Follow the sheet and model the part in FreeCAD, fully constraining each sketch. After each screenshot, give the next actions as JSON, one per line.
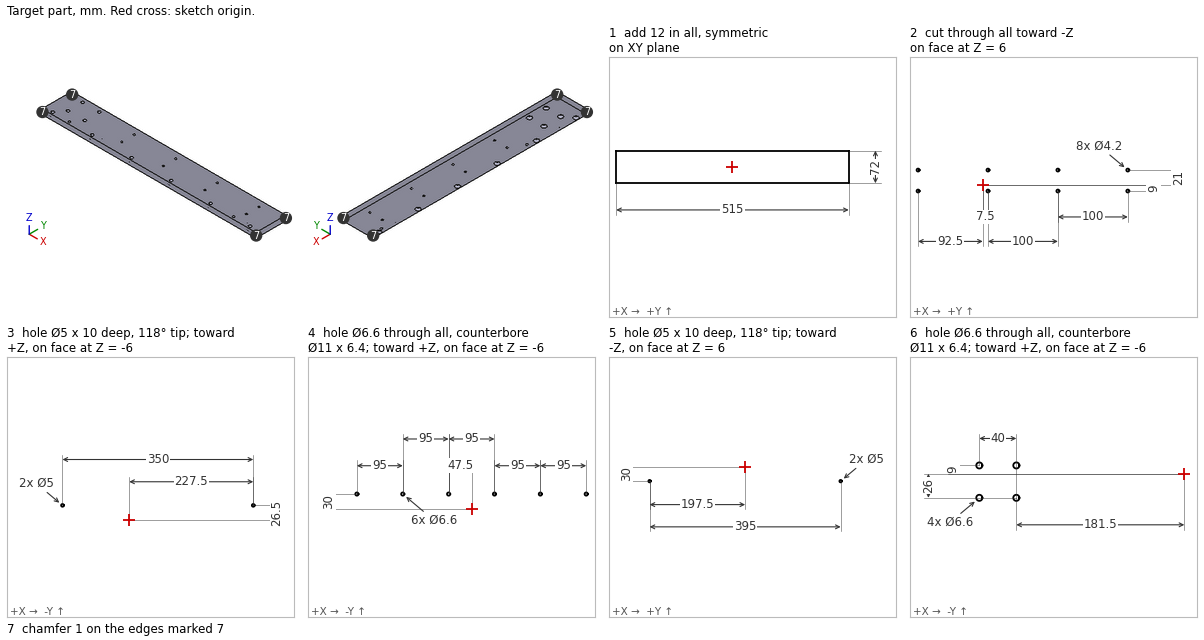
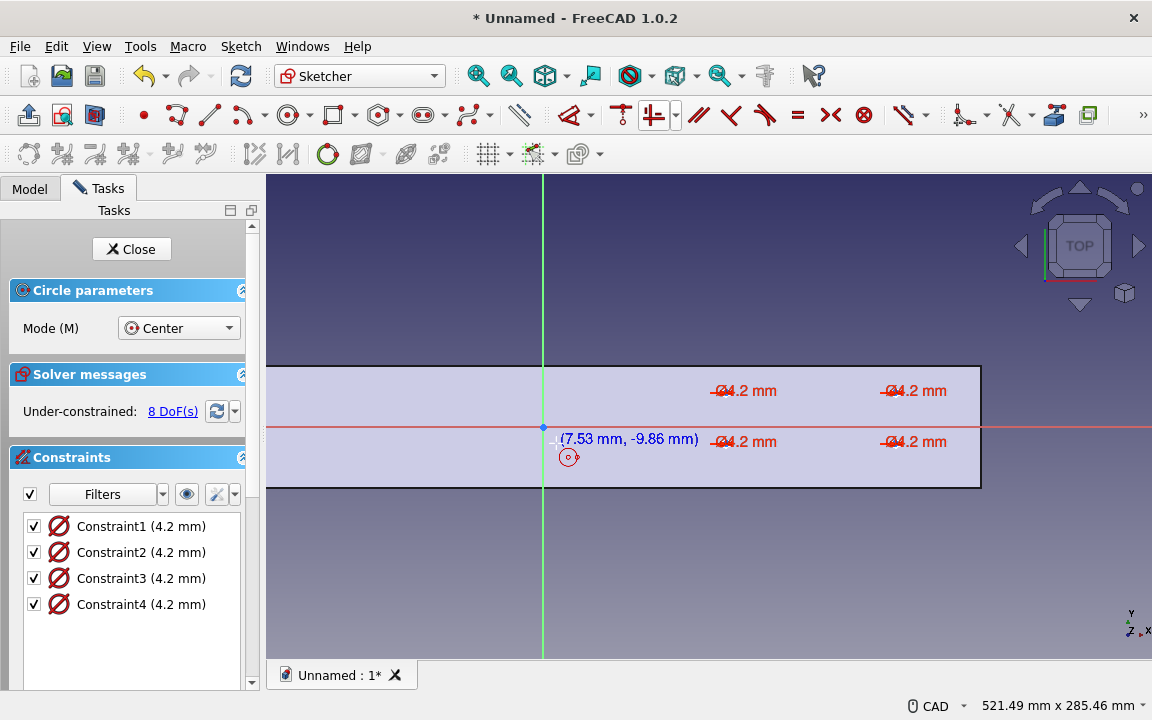
{"action": "scroll", "coordinate": [556, 443], "scroll_direction": "up", "scroll_amount": 2}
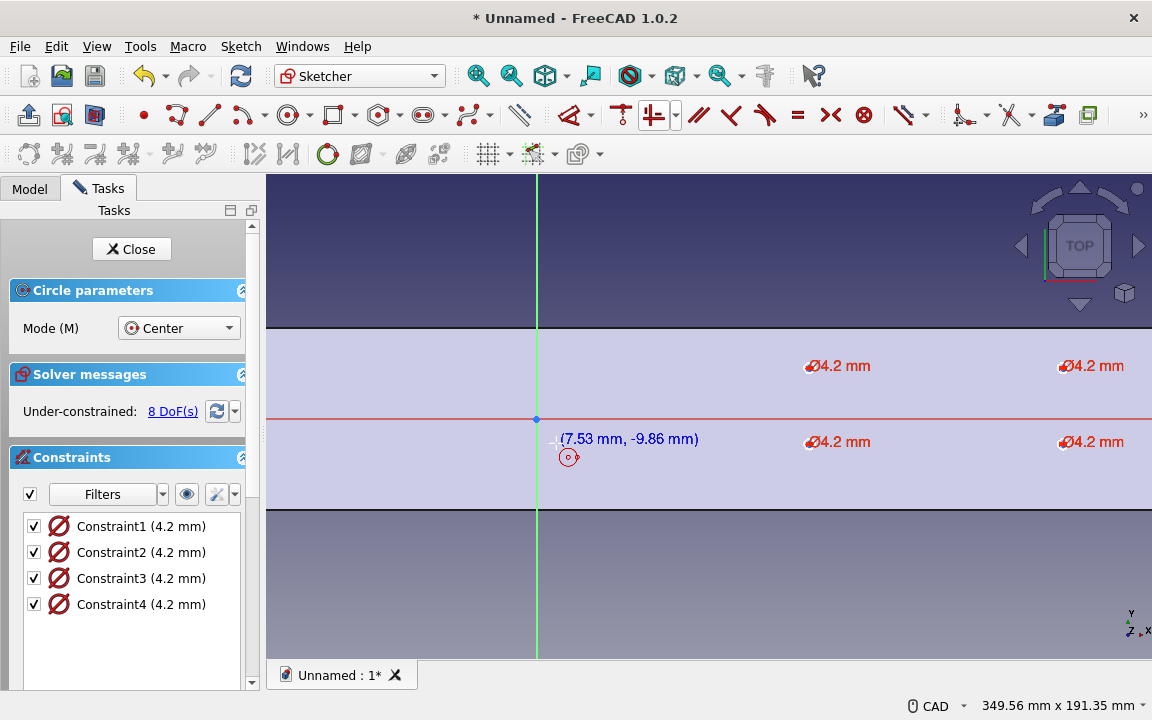
{"action": "left_click", "coordinate": [556, 442]}
{"action": "mouse_move", "coordinate": [560, 438]}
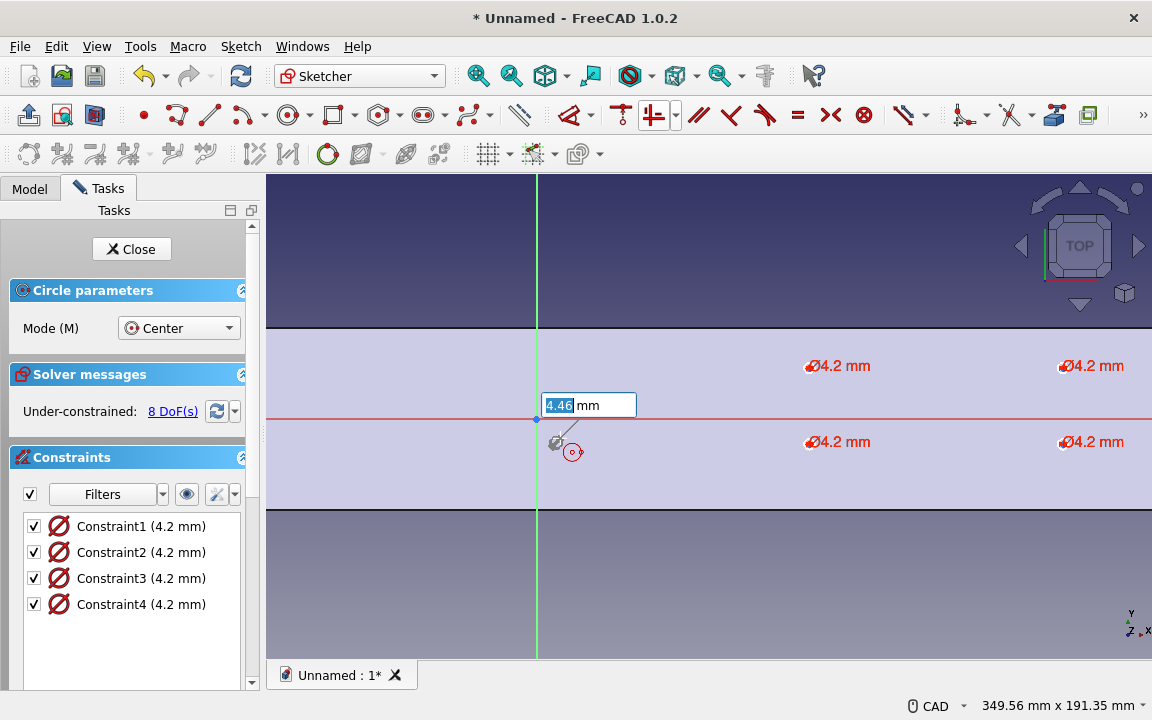
{"action": "type", "text": "4.2"}
{"action": "key", "text": "Return"}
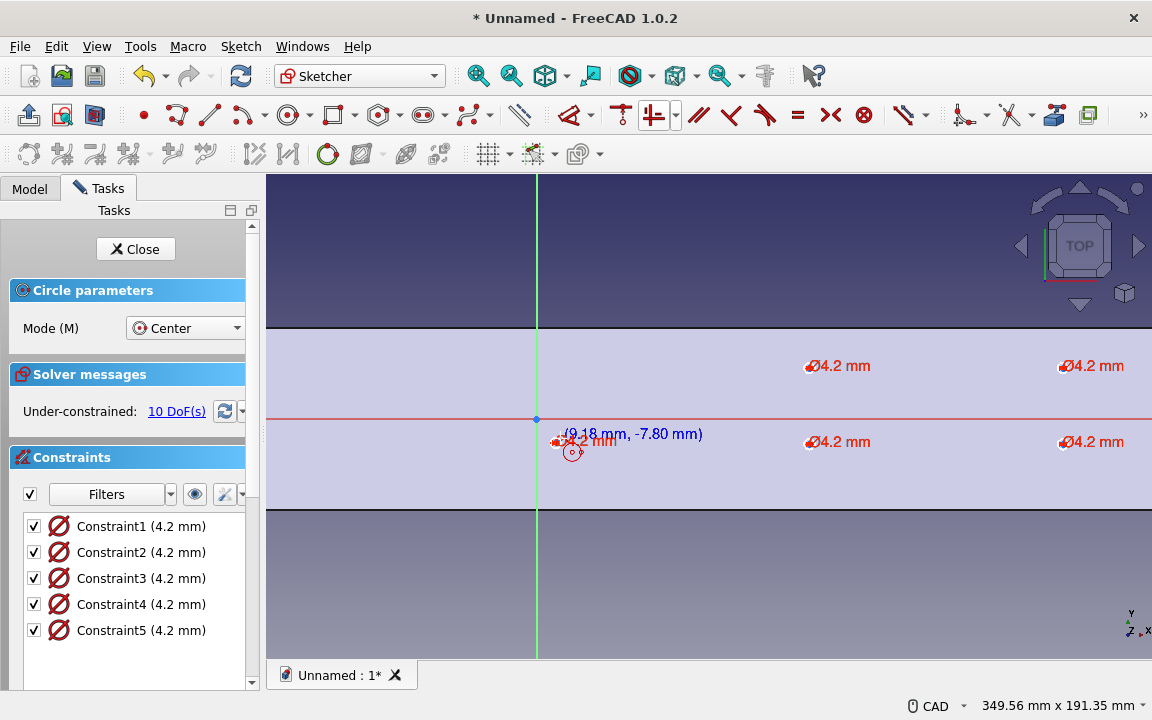
{"action": "scroll", "coordinate": [556, 366], "scroll_direction": "up", "scroll_amount": 8}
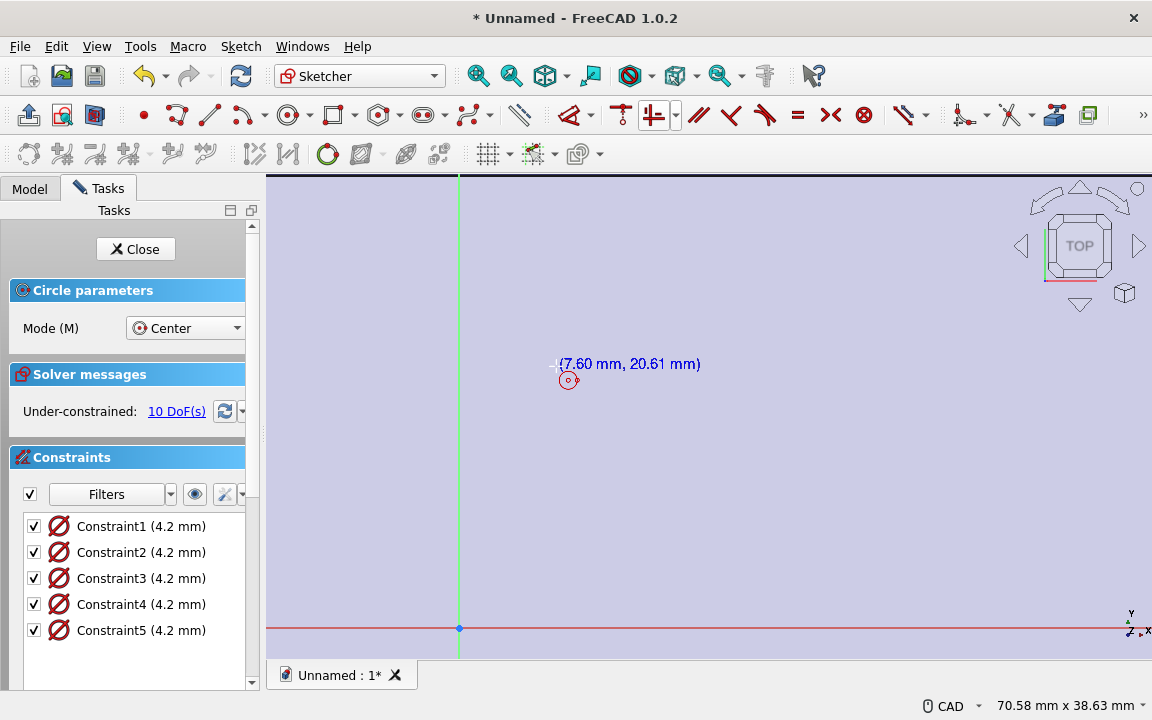
{"action": "scroll", "coordinate": [556, 395], "scroll_direction": "down", "scroll_amount": 10}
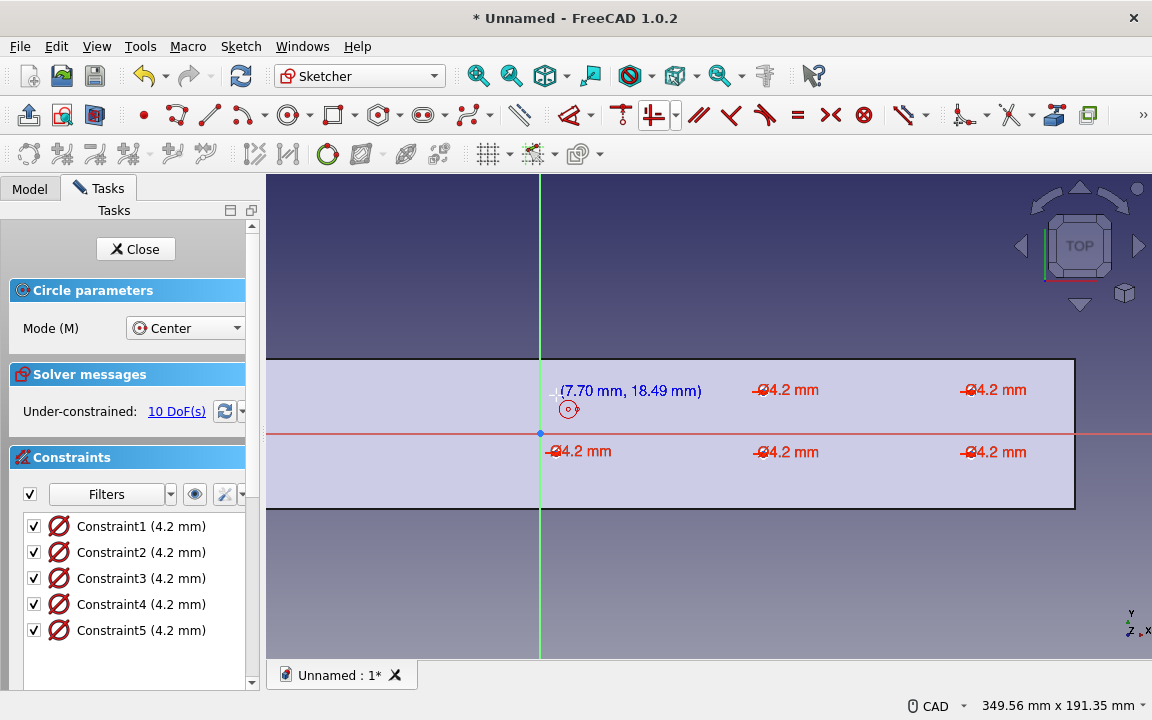
{"action": "scroll", "coordinate": [556, 391], "scroll_direction": "up", "scroll_amount": 2}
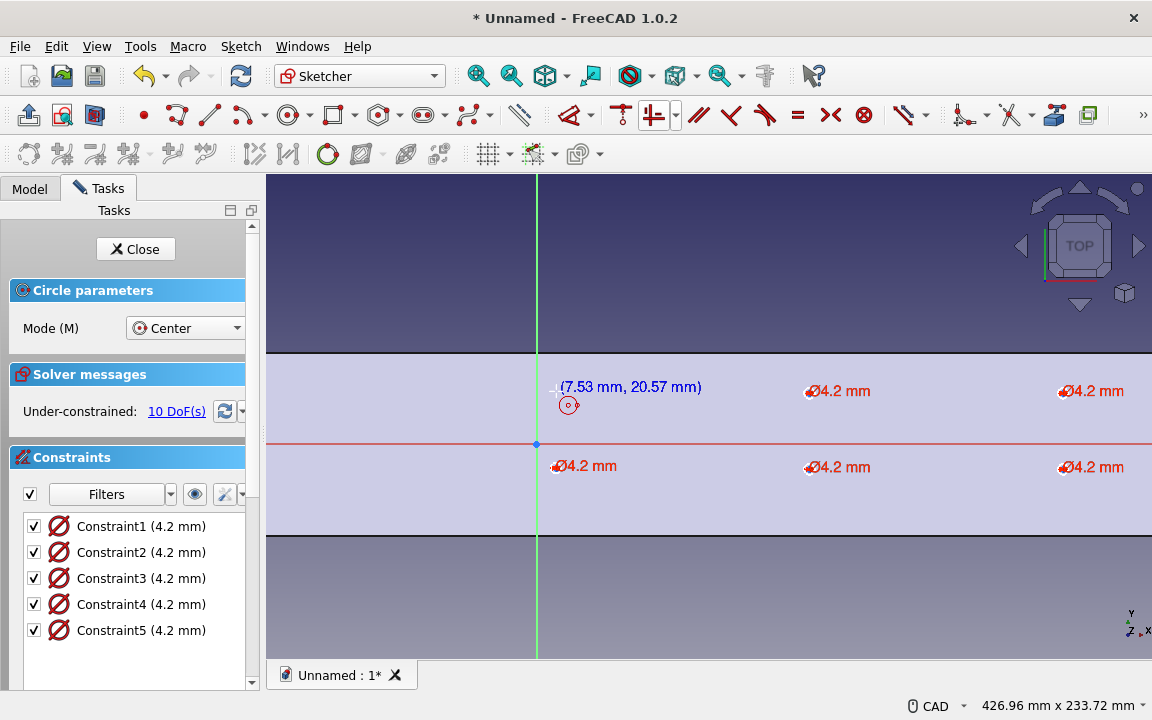
{"action": "left_click", "coordinate": [556, 391]}
{"action": "mouse_move", "coordinate": [560, 387]}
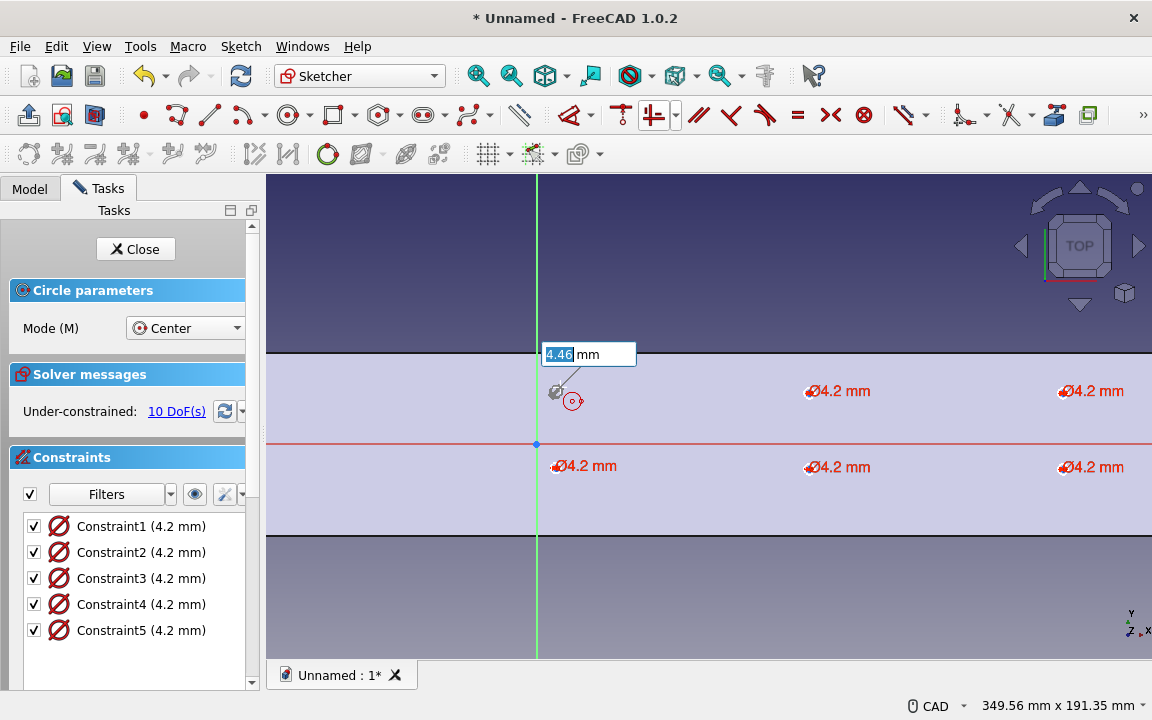
{"action": "type", "text": "4.2"}
{"action": "key", "text": "Return"}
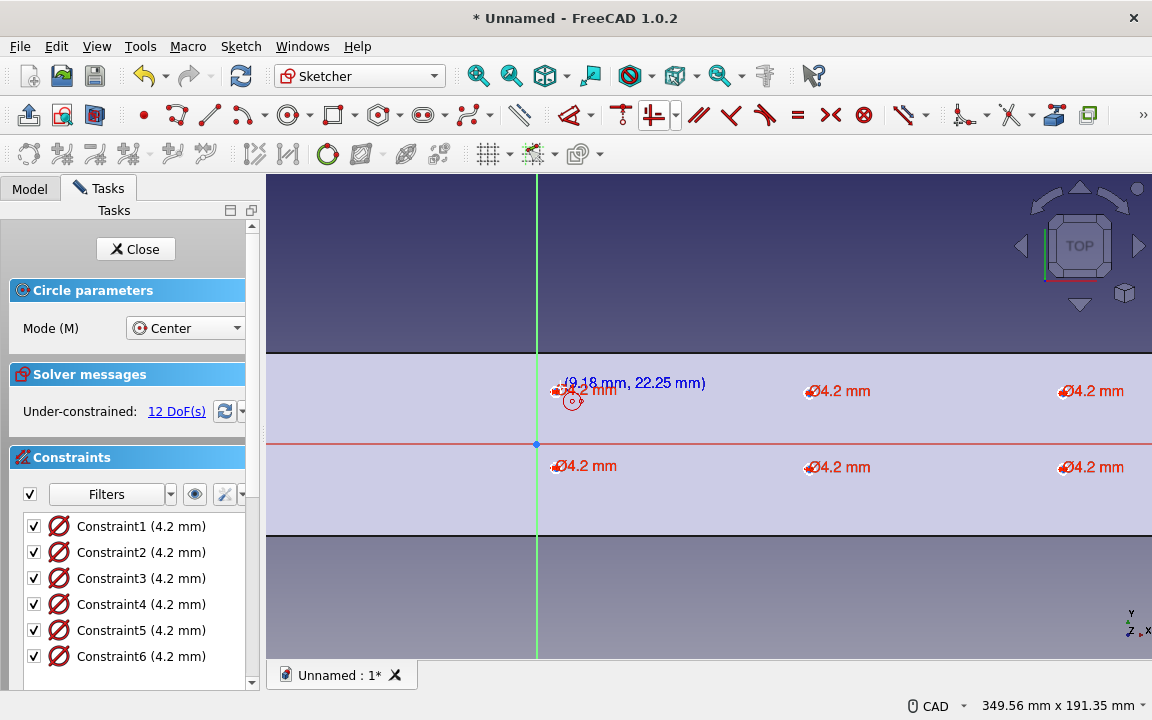
{"action": "scroll", "coordinate": [302, 467], "scroll_direction": "up", "scroll_amount": 8}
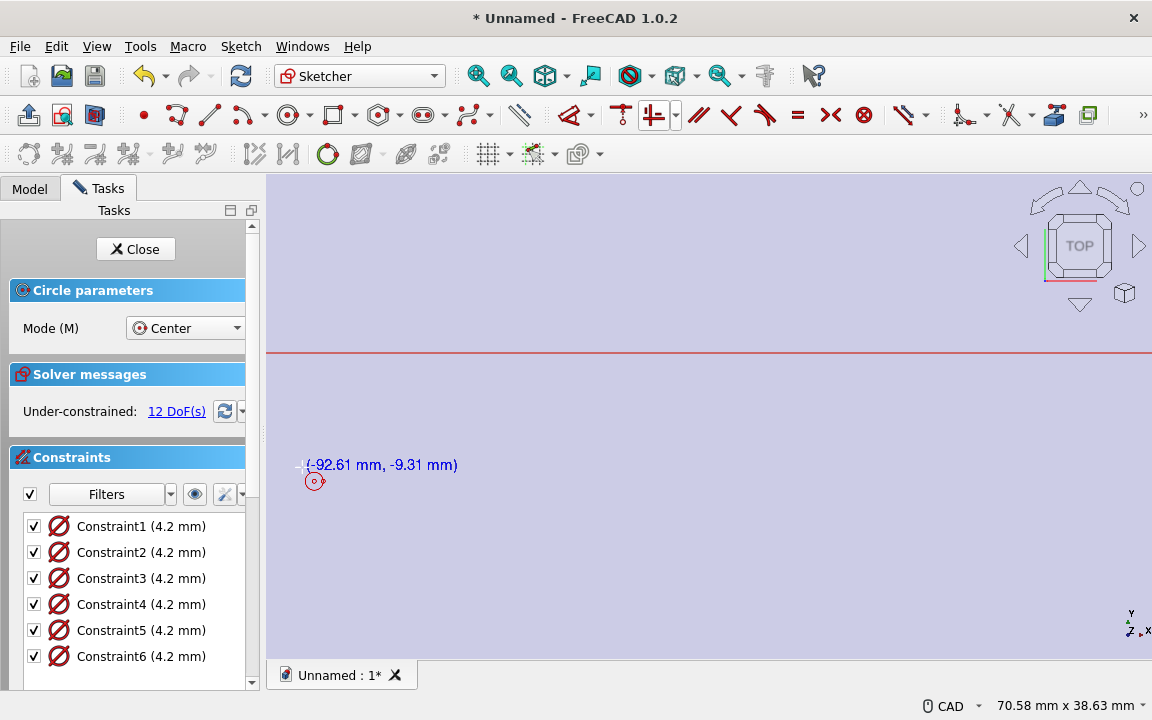
{"action": "scroll", "coordinate": [399, 438], "scroll_direction": "down", "scroll_amount": 10}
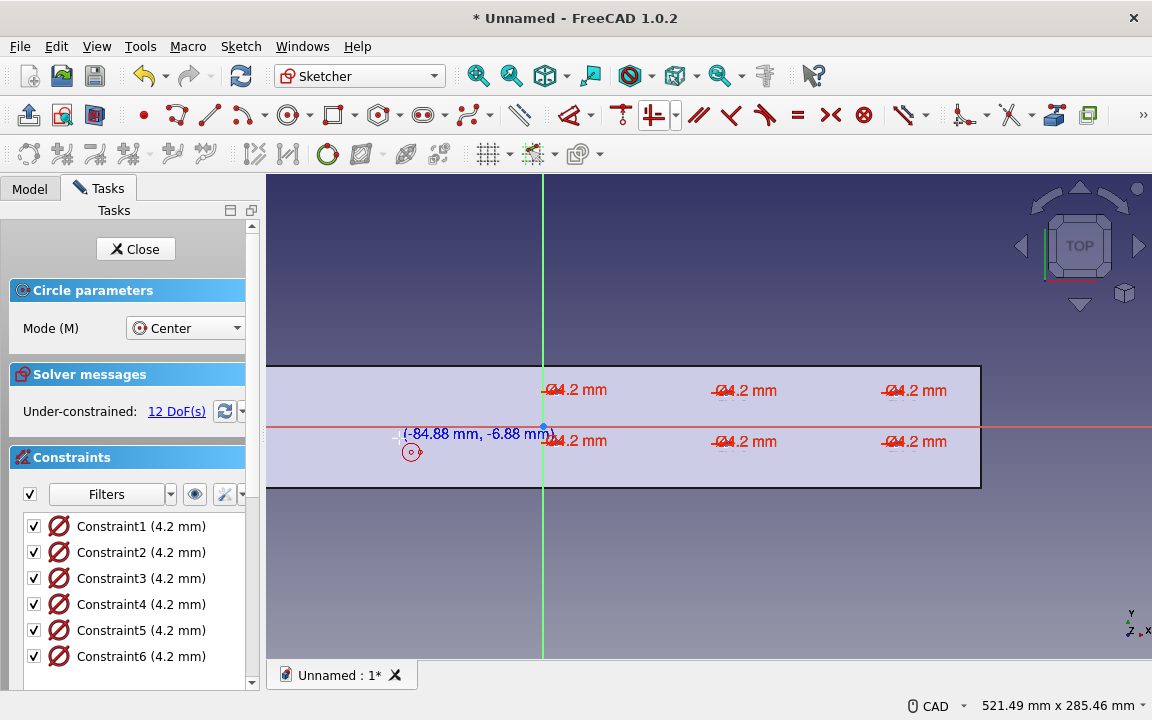
{"action": "left_click", "coordinate": [386, 442]}
{"action": "mouse_move", "coordinate": [389, 445]}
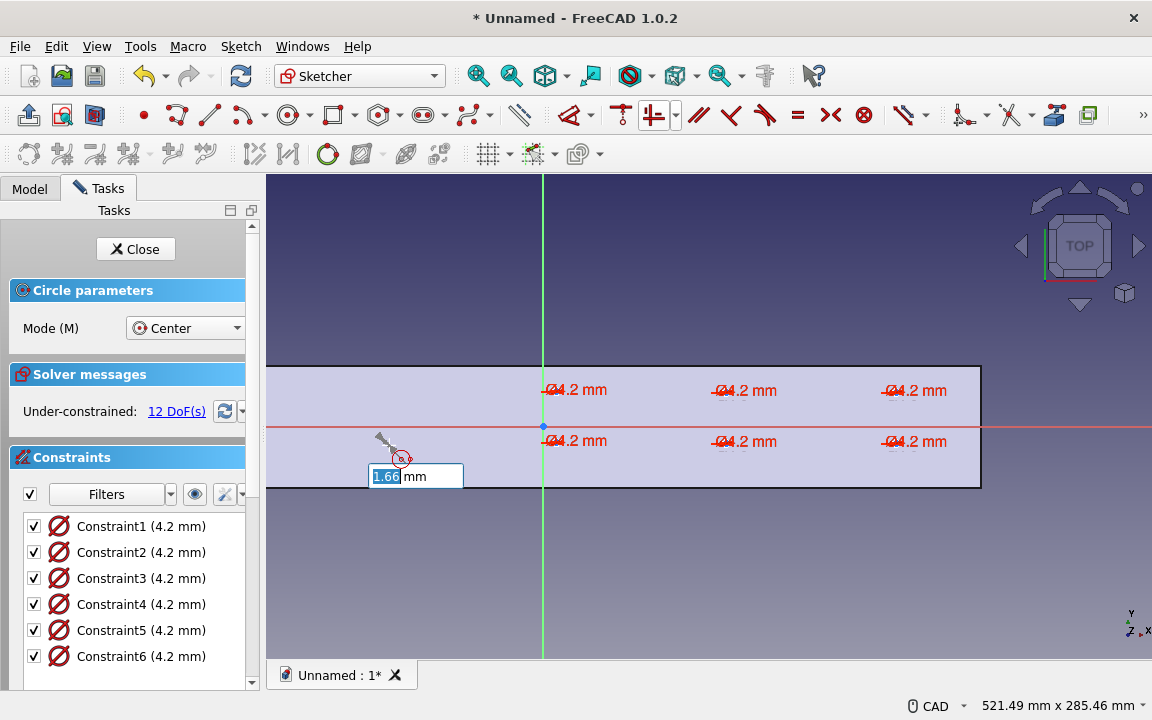
{"action": "type", "text": "4.2"}
{"action": "key", "text": "Return"}